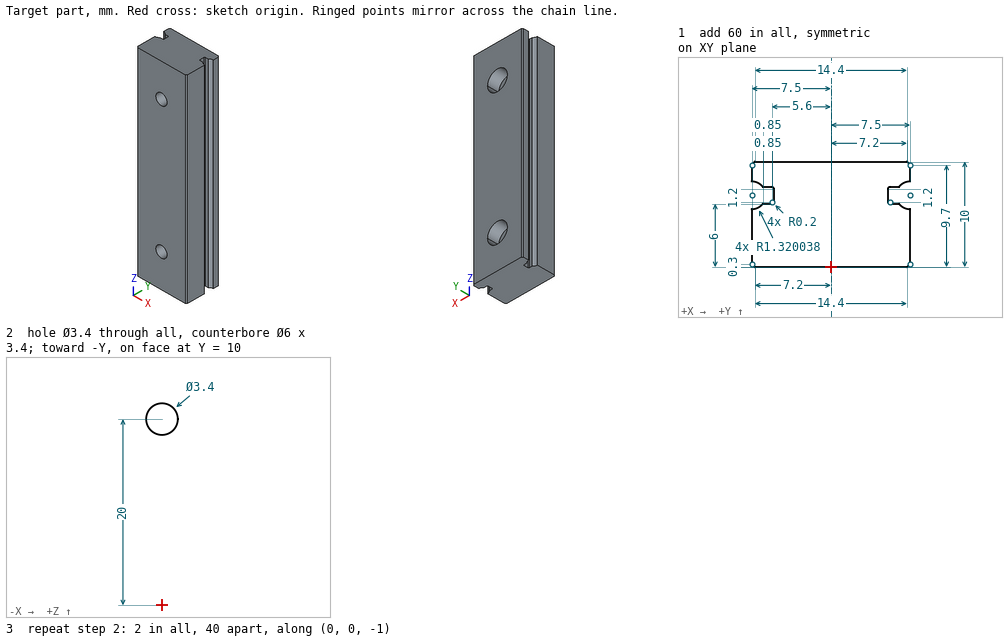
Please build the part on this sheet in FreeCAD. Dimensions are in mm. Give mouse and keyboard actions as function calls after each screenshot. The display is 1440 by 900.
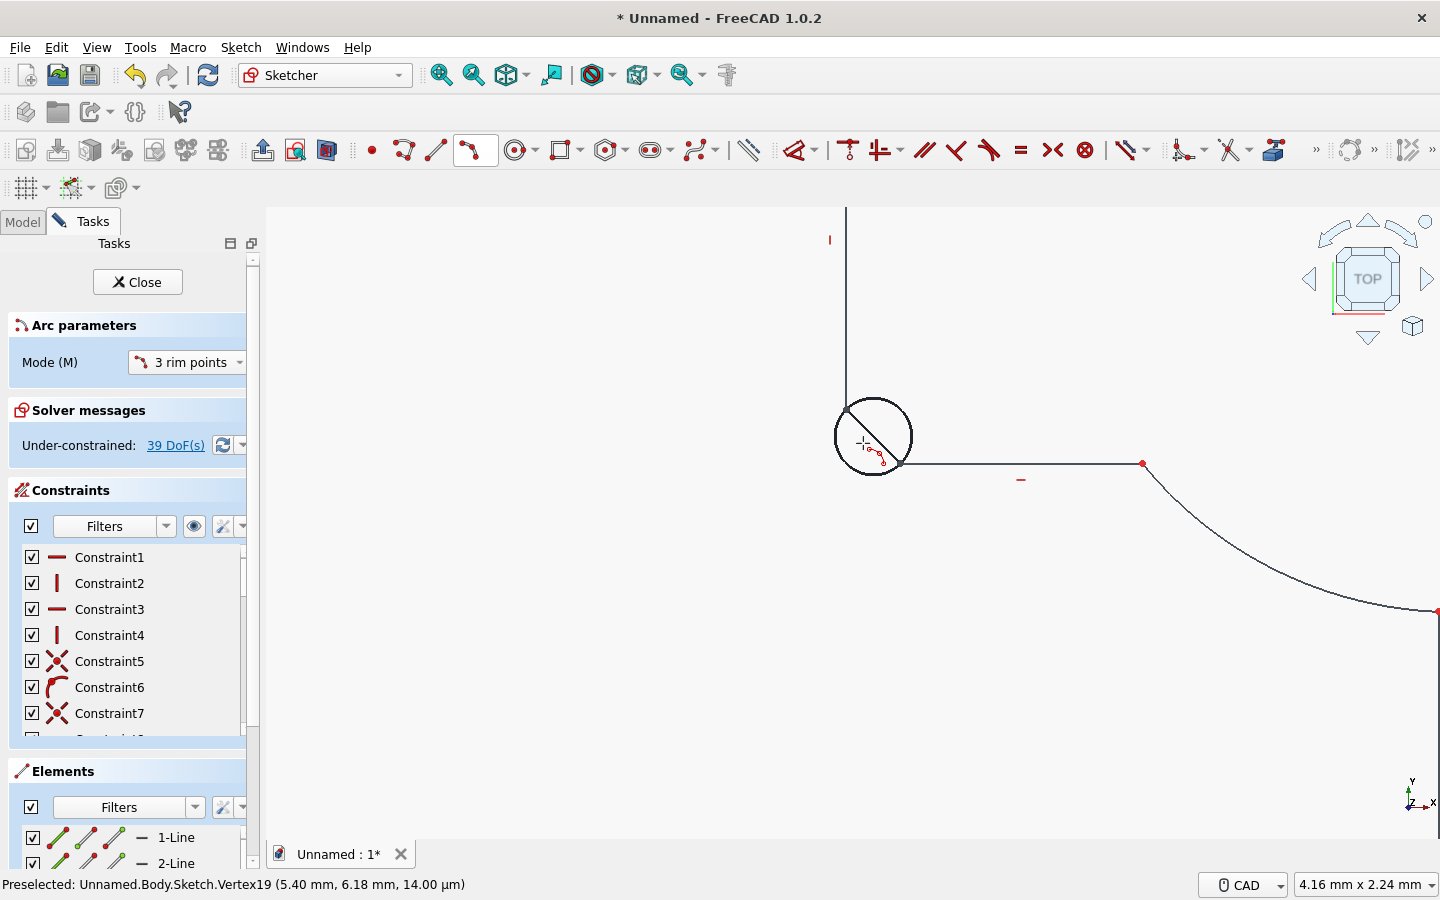
click(863, 443)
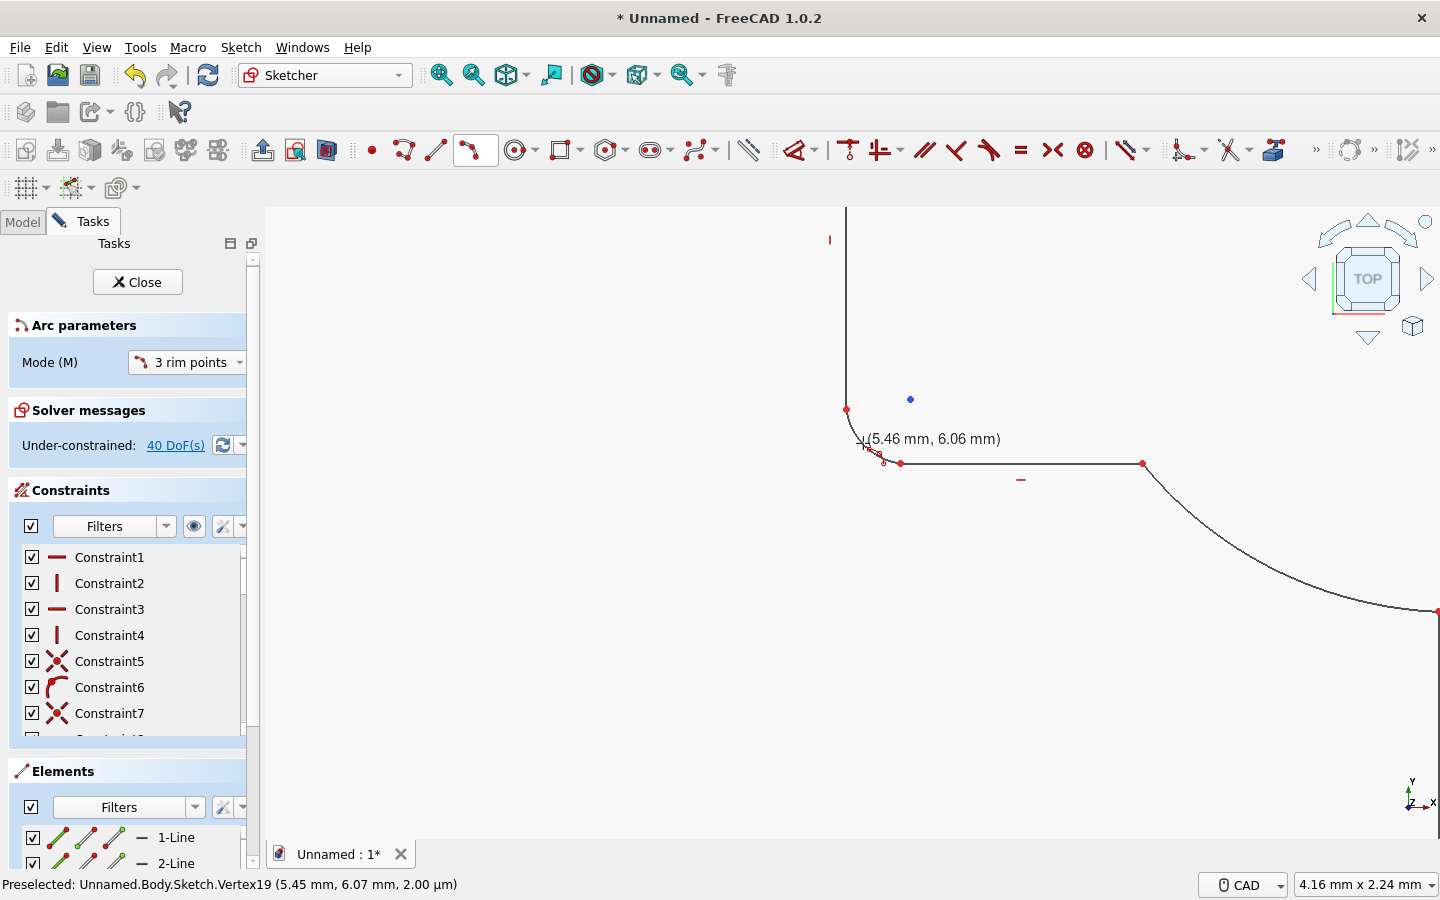
scroll(1014, 489, down, 10)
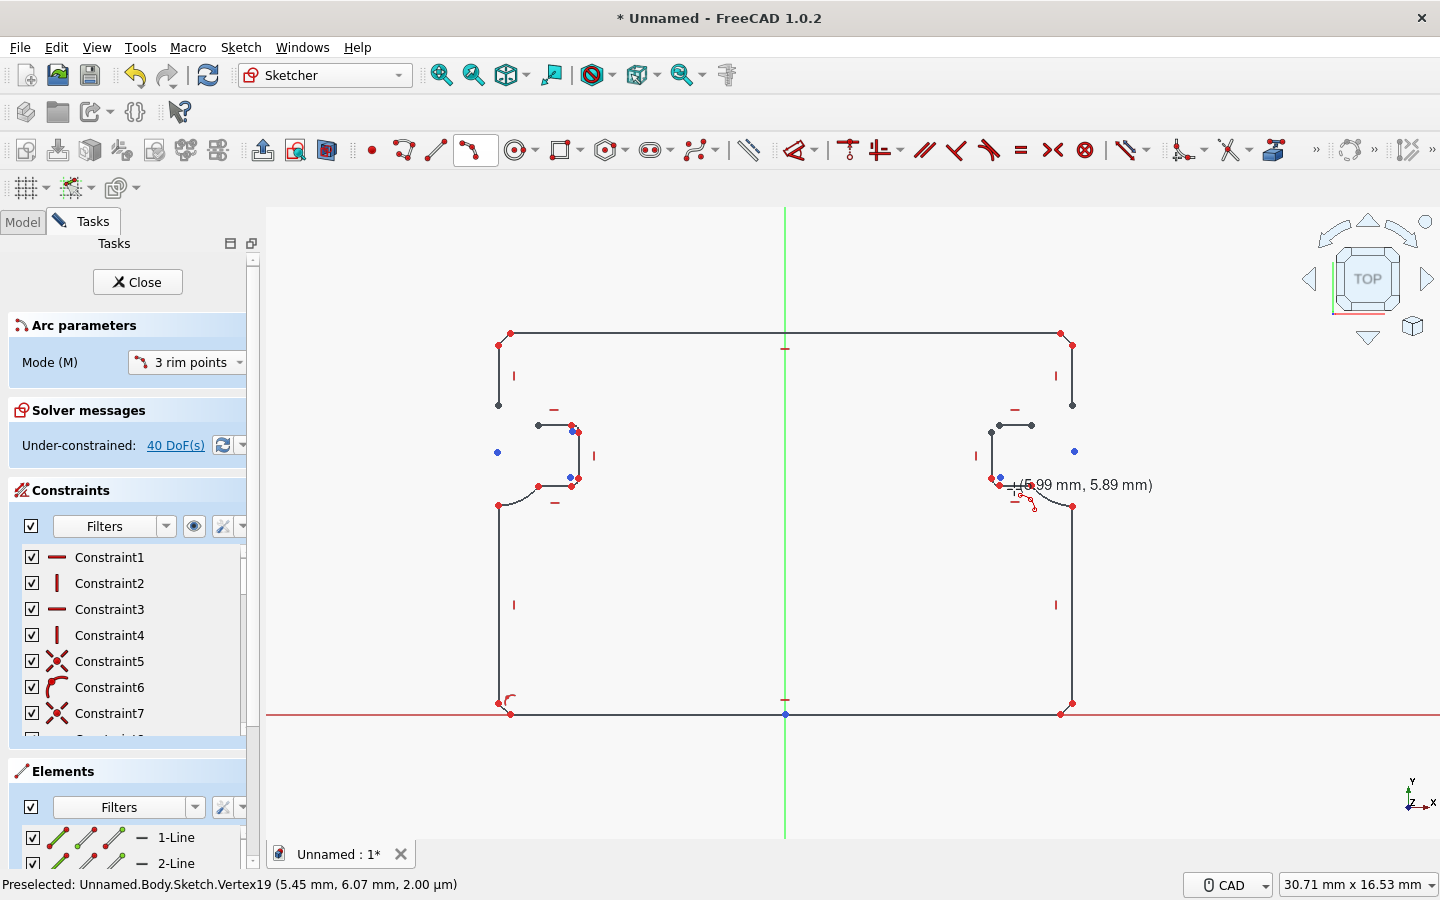
scroll(992, 432, up, 2)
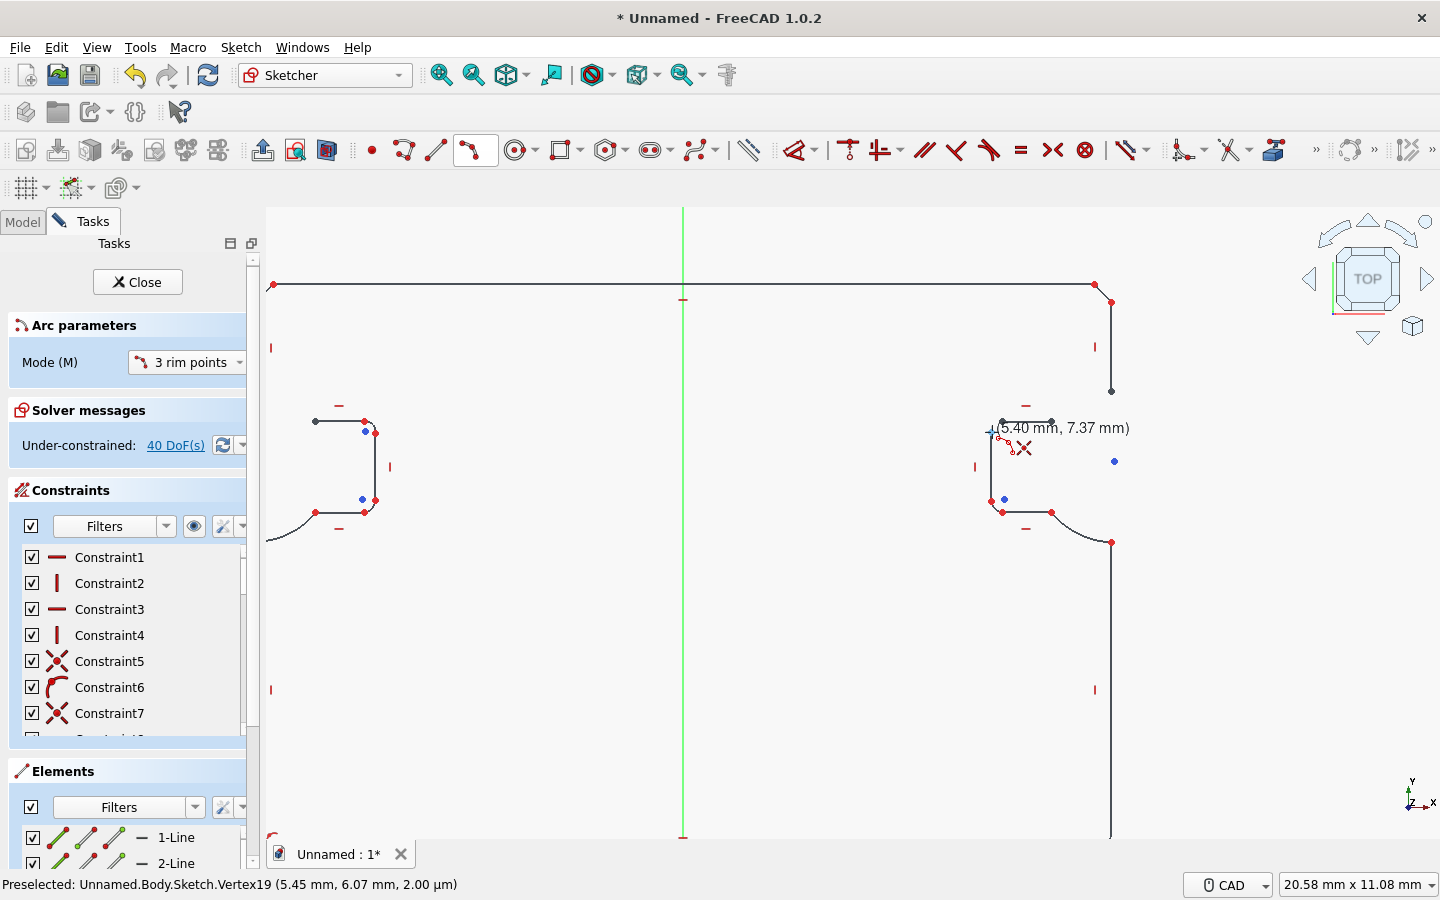
click(991, 433)
click(1002, 422)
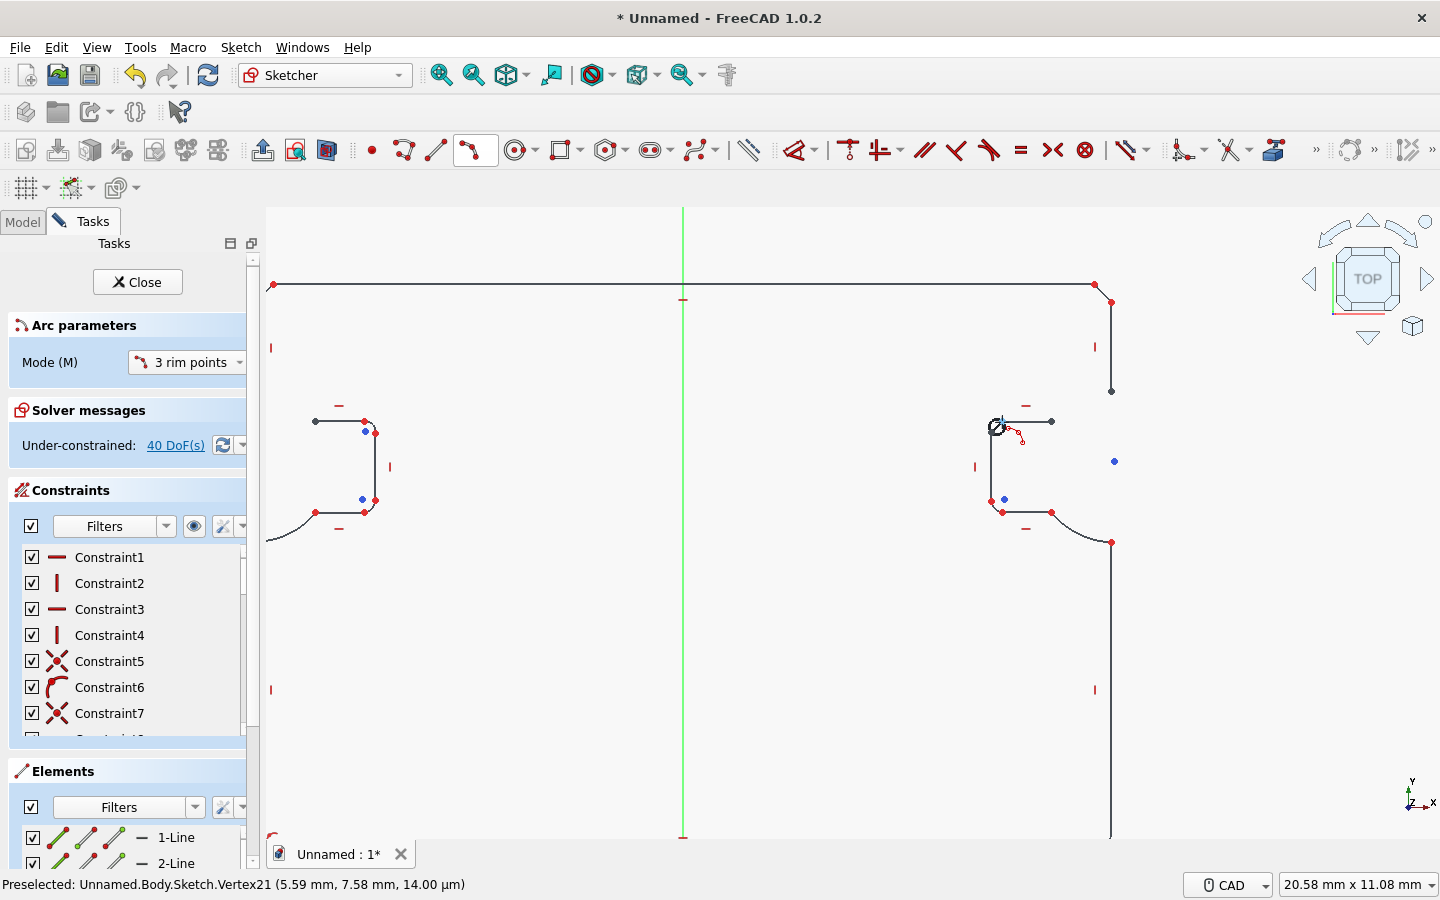
scroll(995, 424, up, 8)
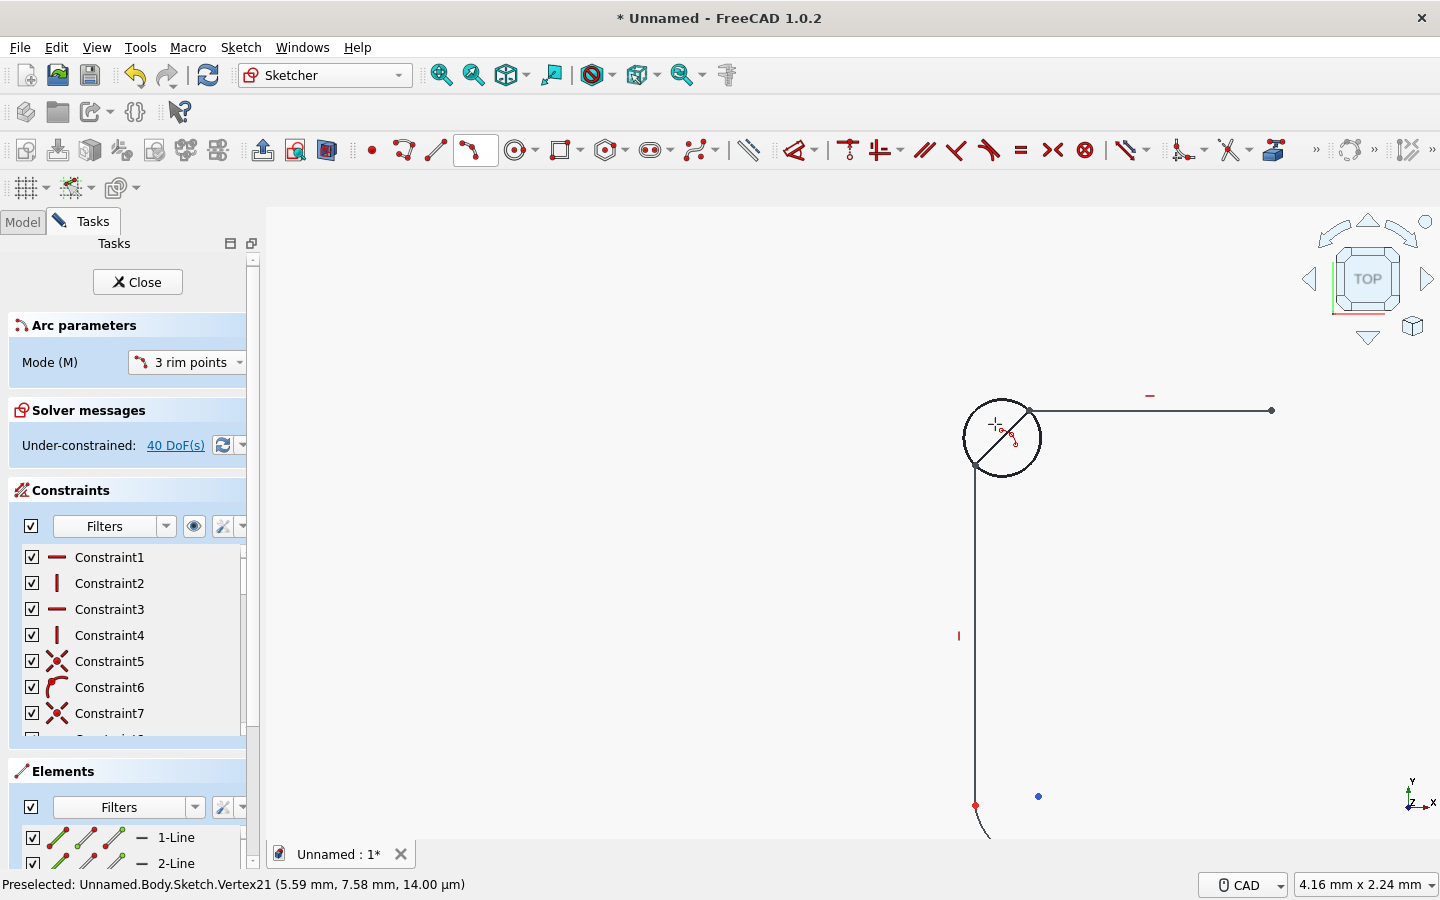
click(992, 421)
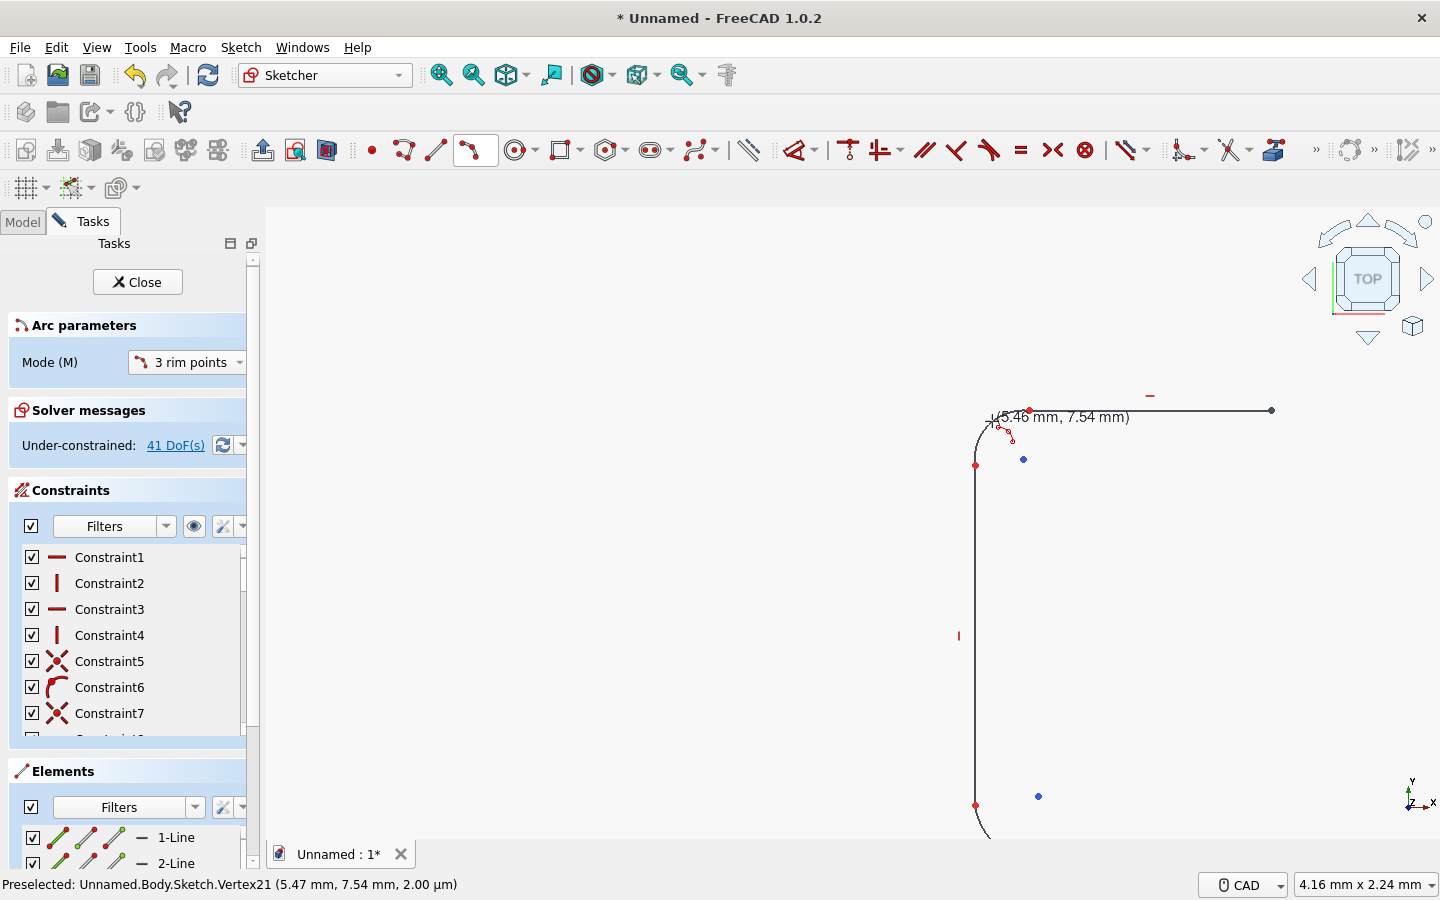
scroll(993, 427, down, 10)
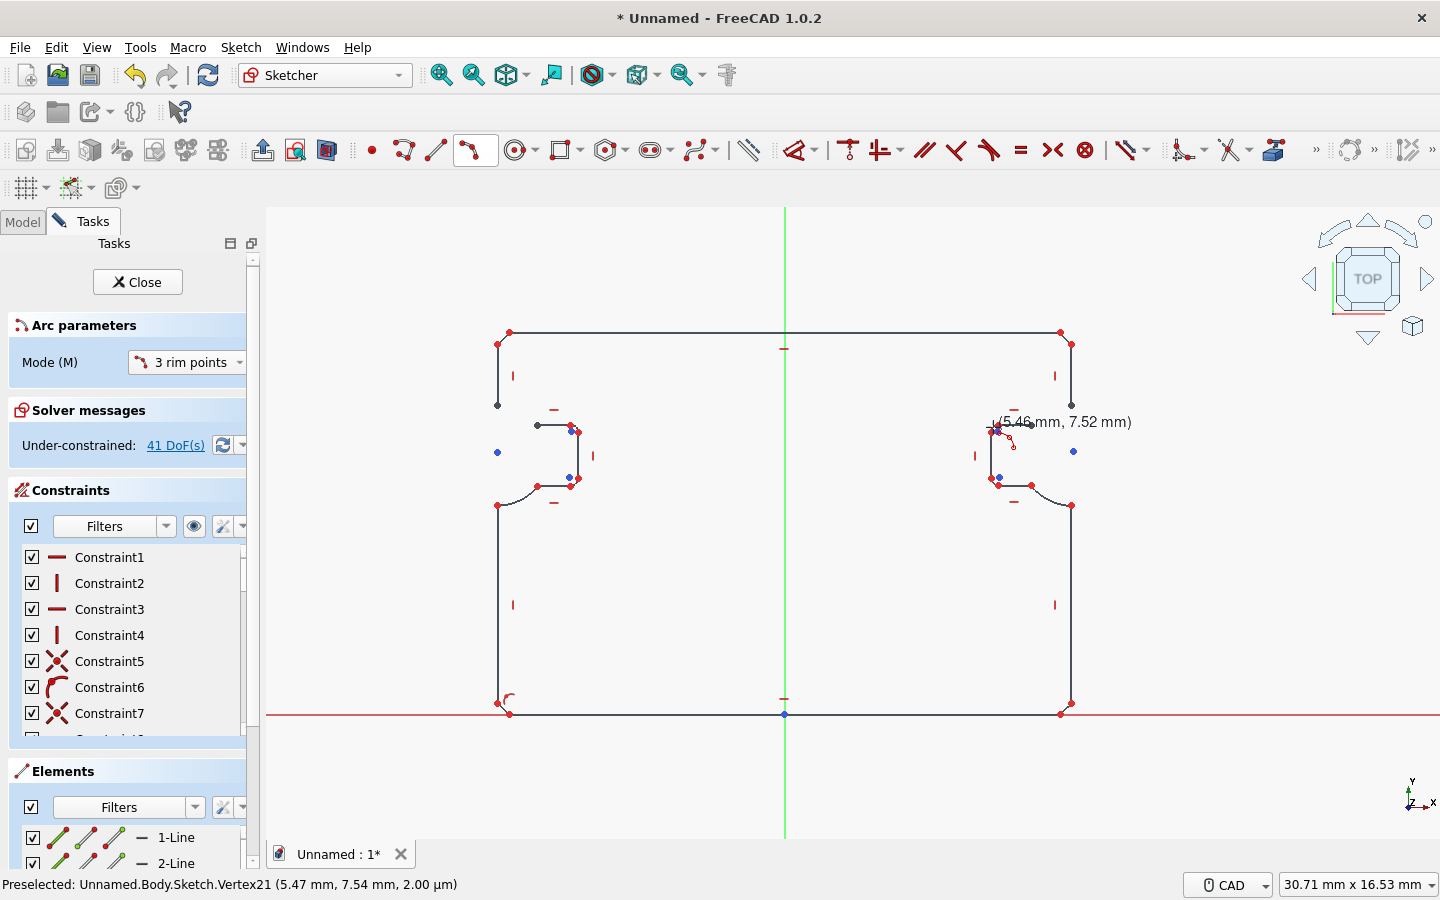
click(1031, 425)
click(1071, 405)